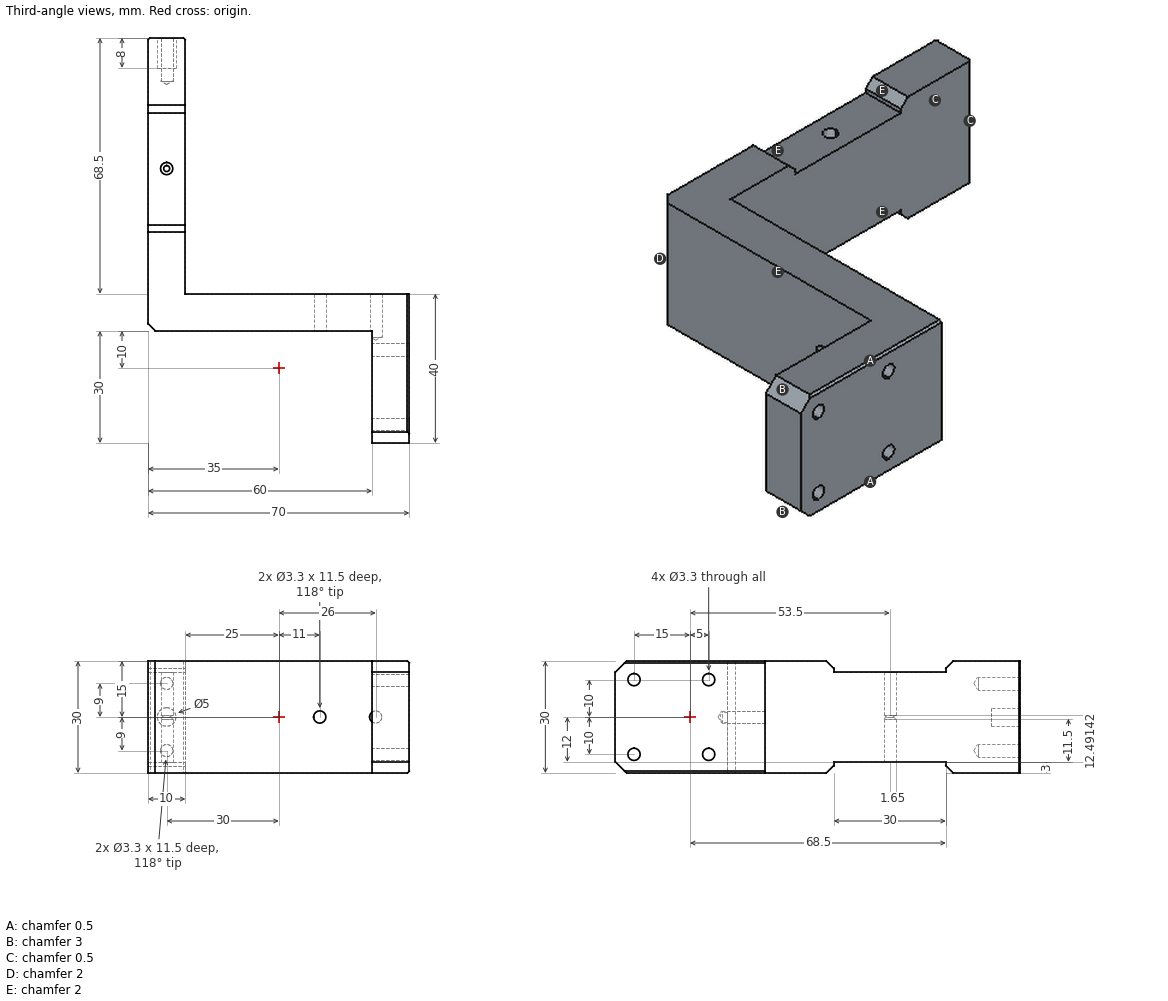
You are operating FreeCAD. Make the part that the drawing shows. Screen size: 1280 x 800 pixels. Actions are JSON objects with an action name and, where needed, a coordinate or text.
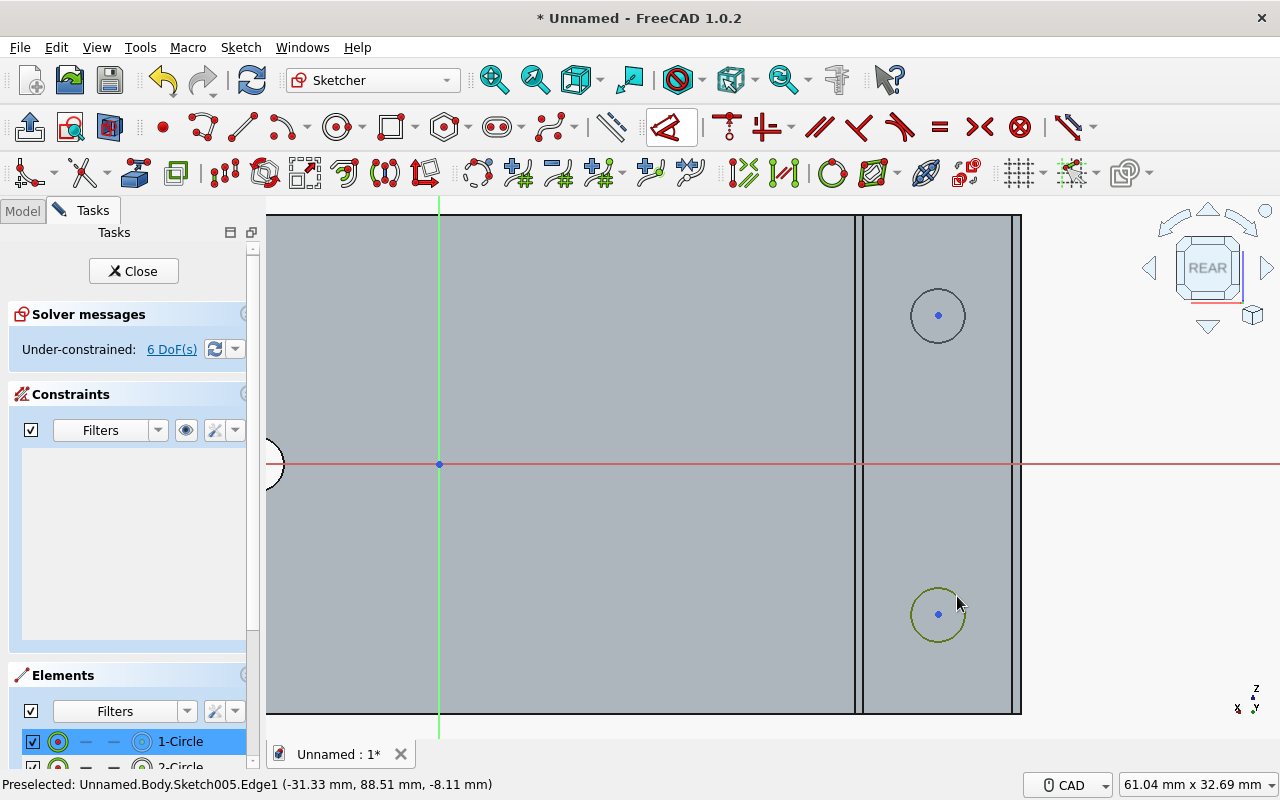
{"action": "left_click", "coordinate": [957, 297]}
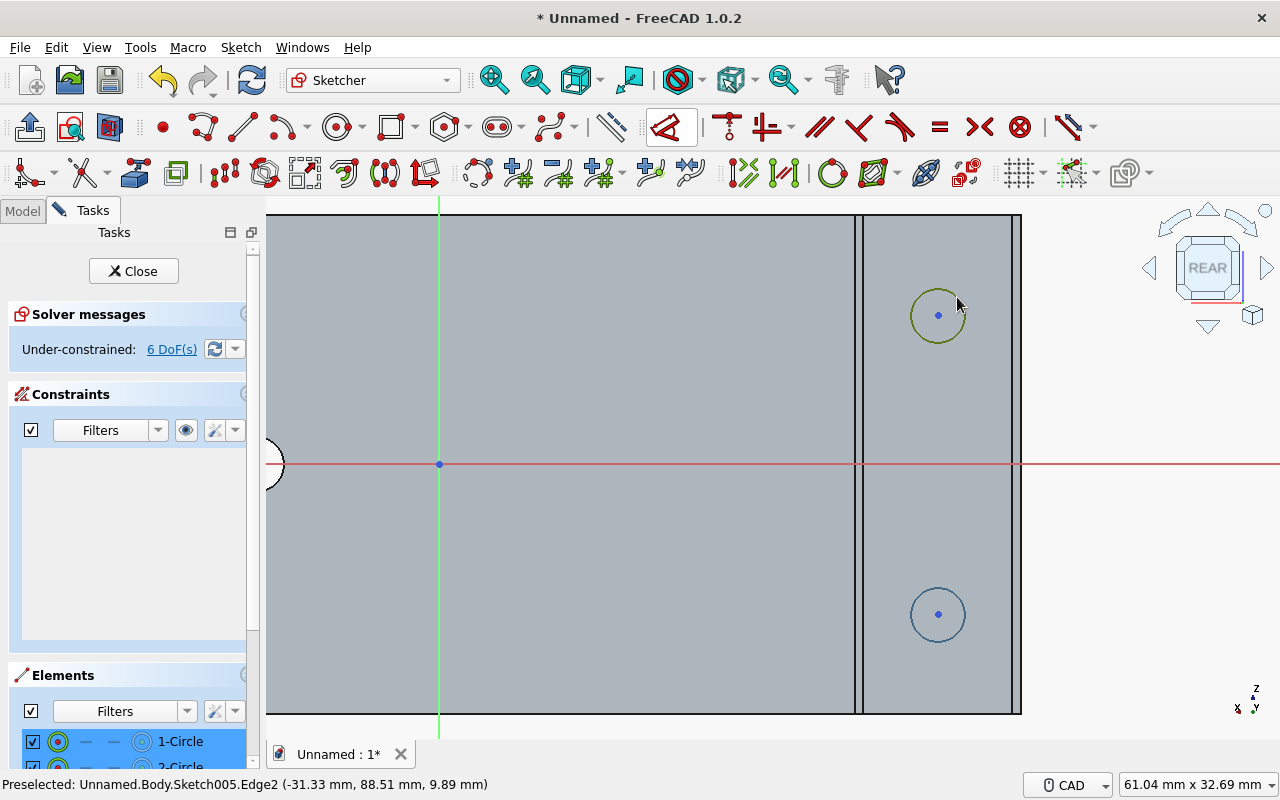
{"action": "left_click", "coordinate": [940, 128]}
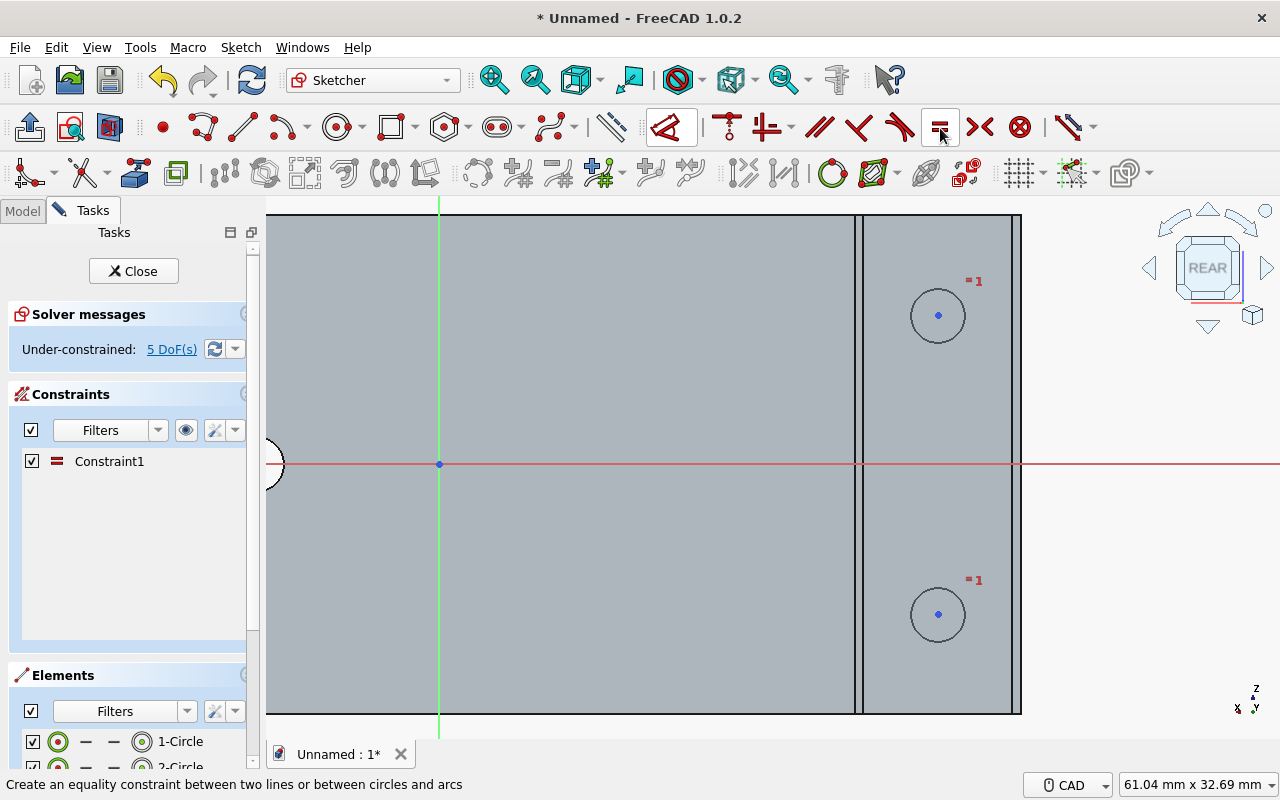
{"action": "left_click", "coordinate": [957, 596]}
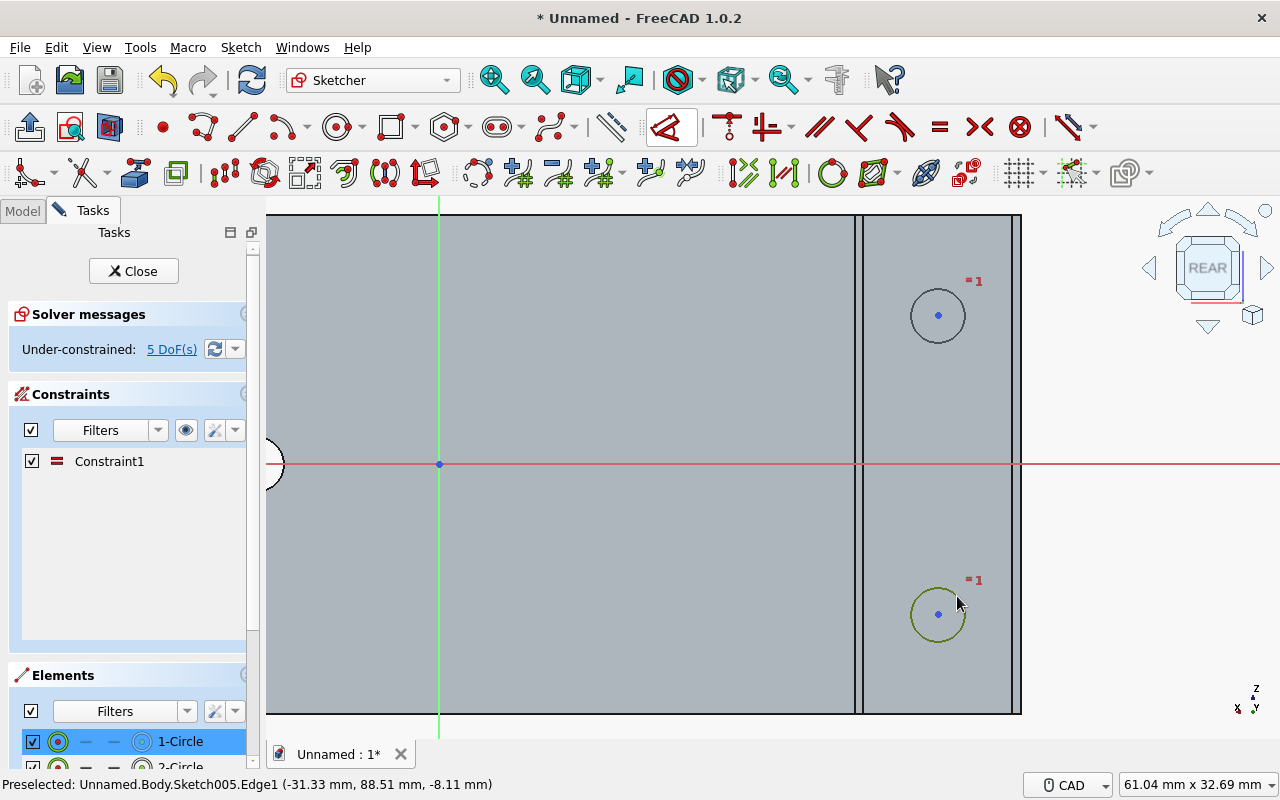
{"action": "key", "text": "k o"}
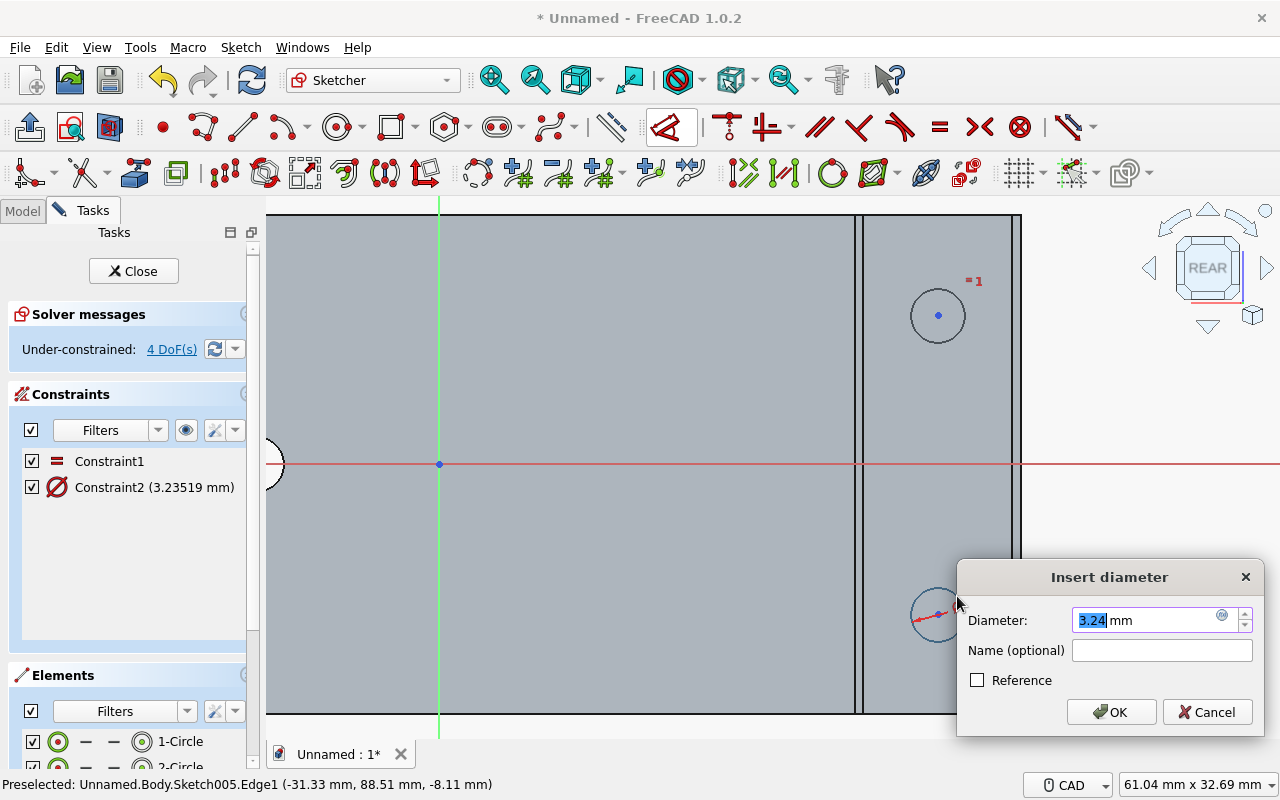
{"action": "type", "text": "3.3"}
{"action": "key", "text": "Return"}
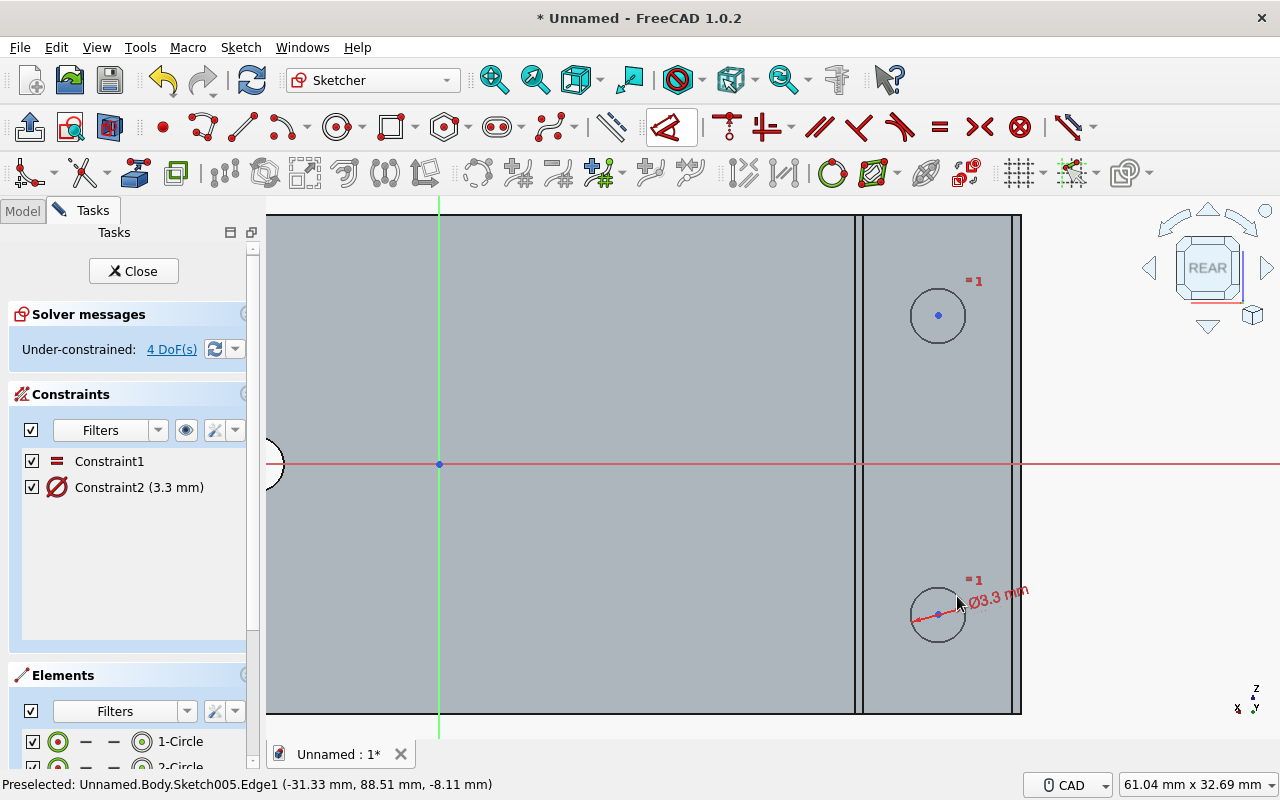
{"action": "left_click", "coordinate": [938, 615]}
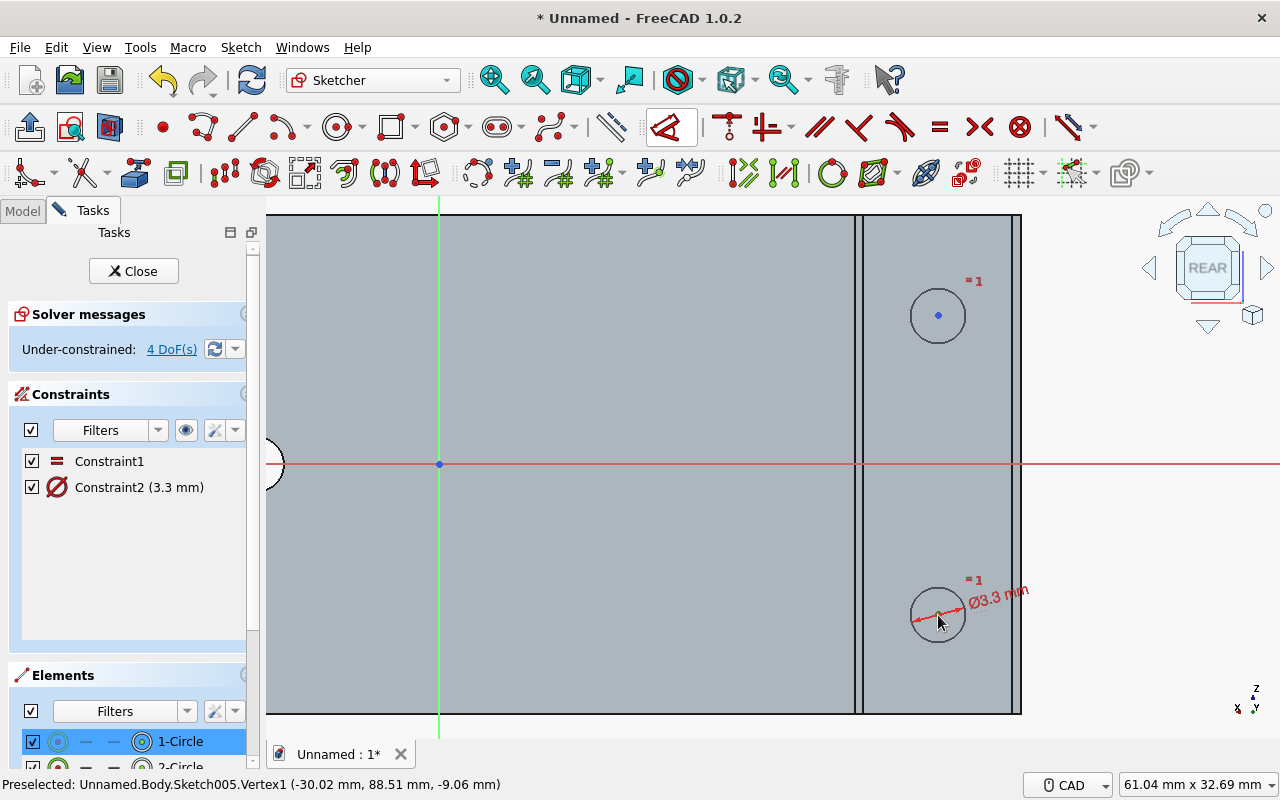
{"action": "left_click", "coordinate": [692, 128]}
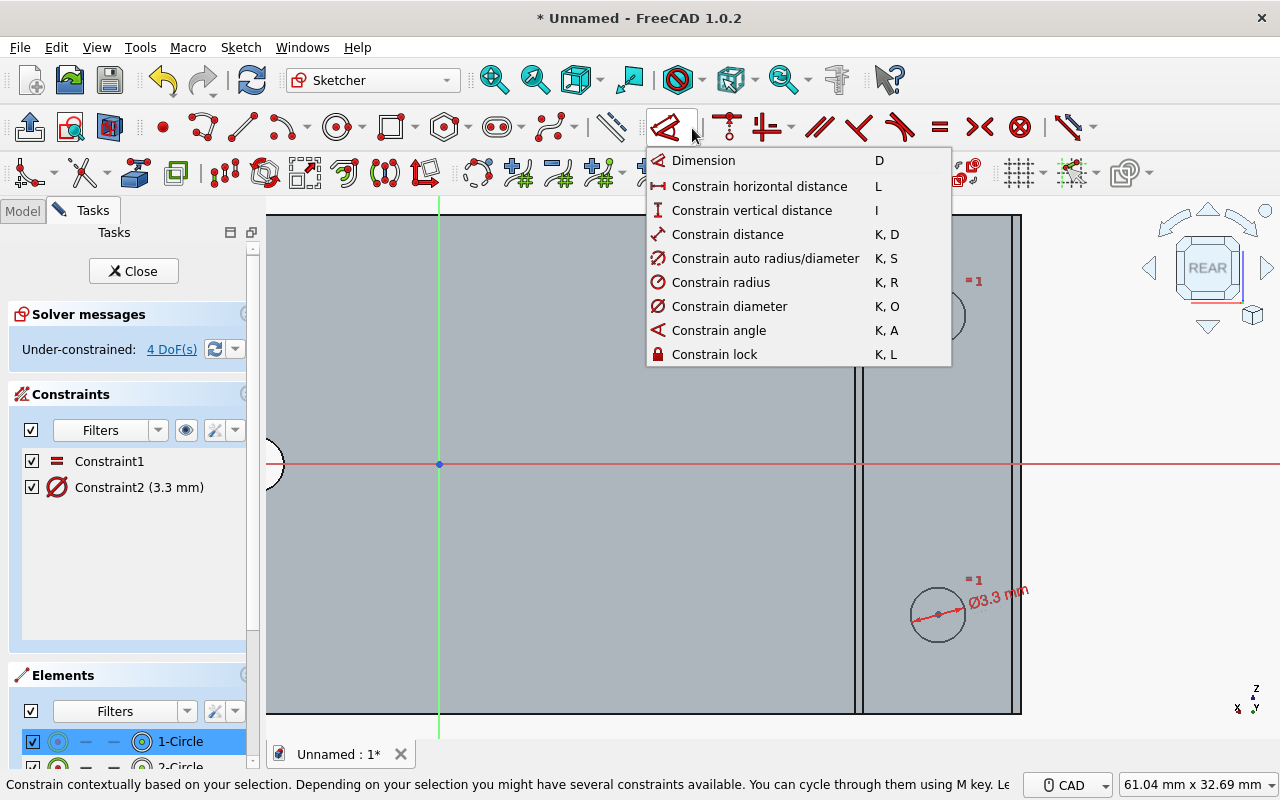
{"action": "left_click", "coordinate": [799, 210]}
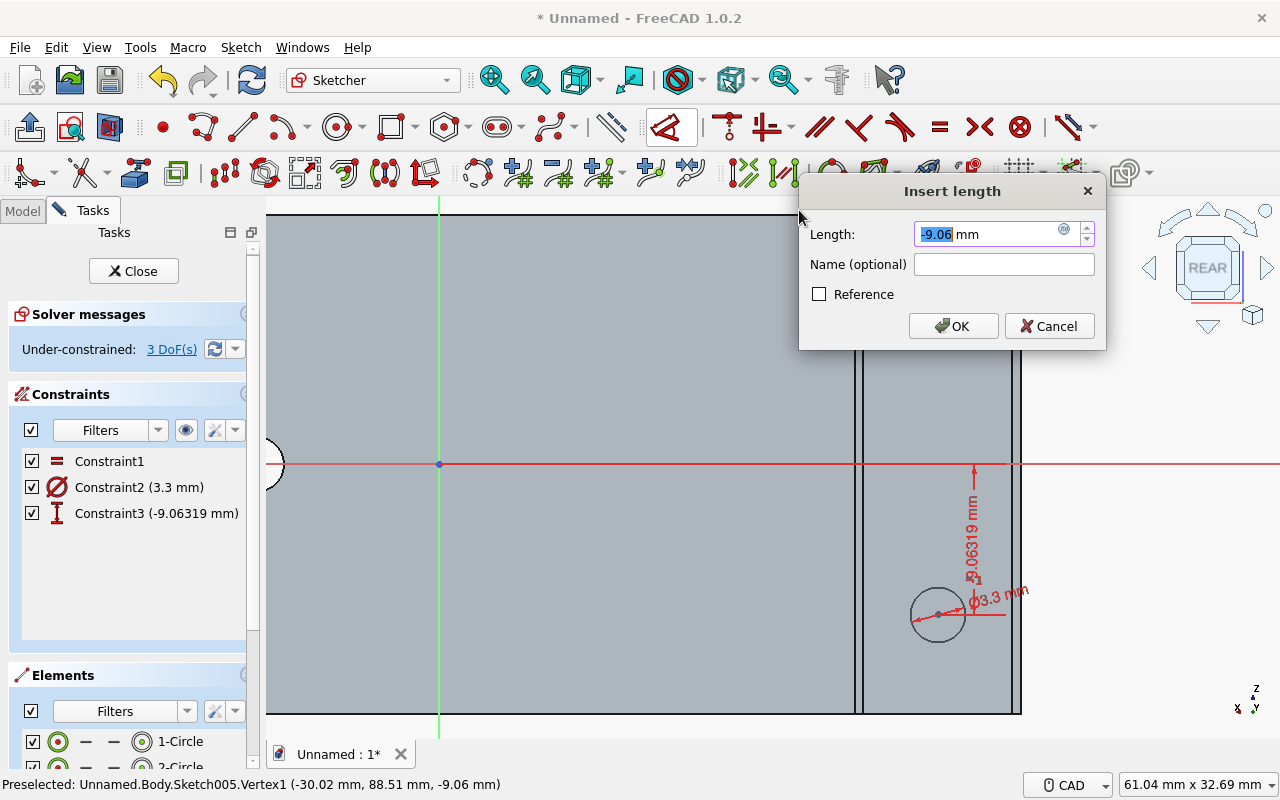
{"action": "type", "text": "-9"}
{"action": "key", "text": "Return"}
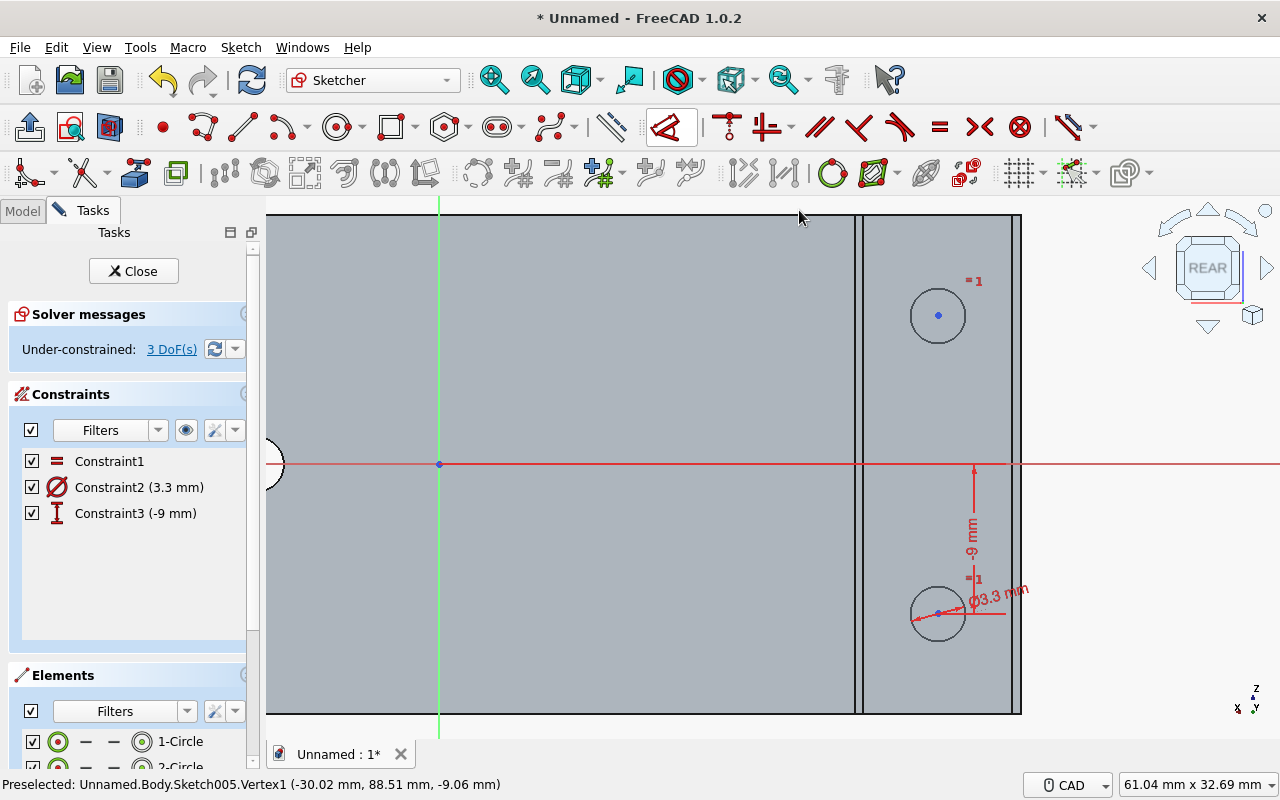
{"action": "left_click", "coordinate": [938, 316]}